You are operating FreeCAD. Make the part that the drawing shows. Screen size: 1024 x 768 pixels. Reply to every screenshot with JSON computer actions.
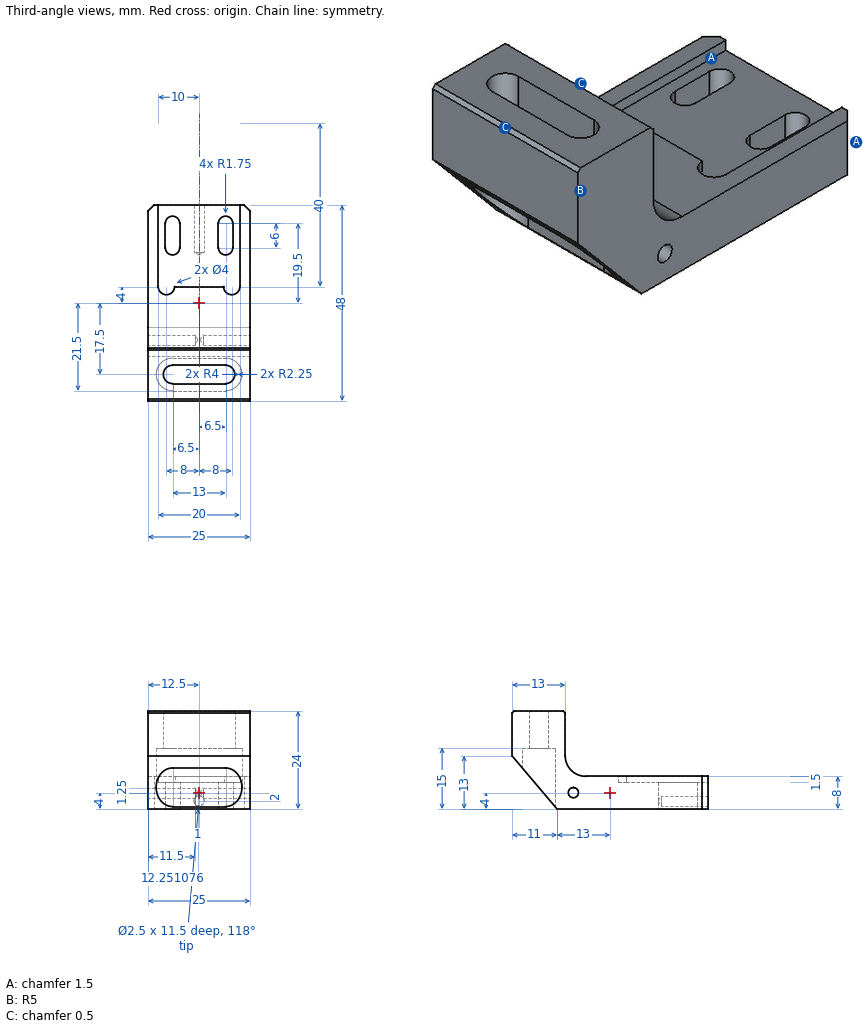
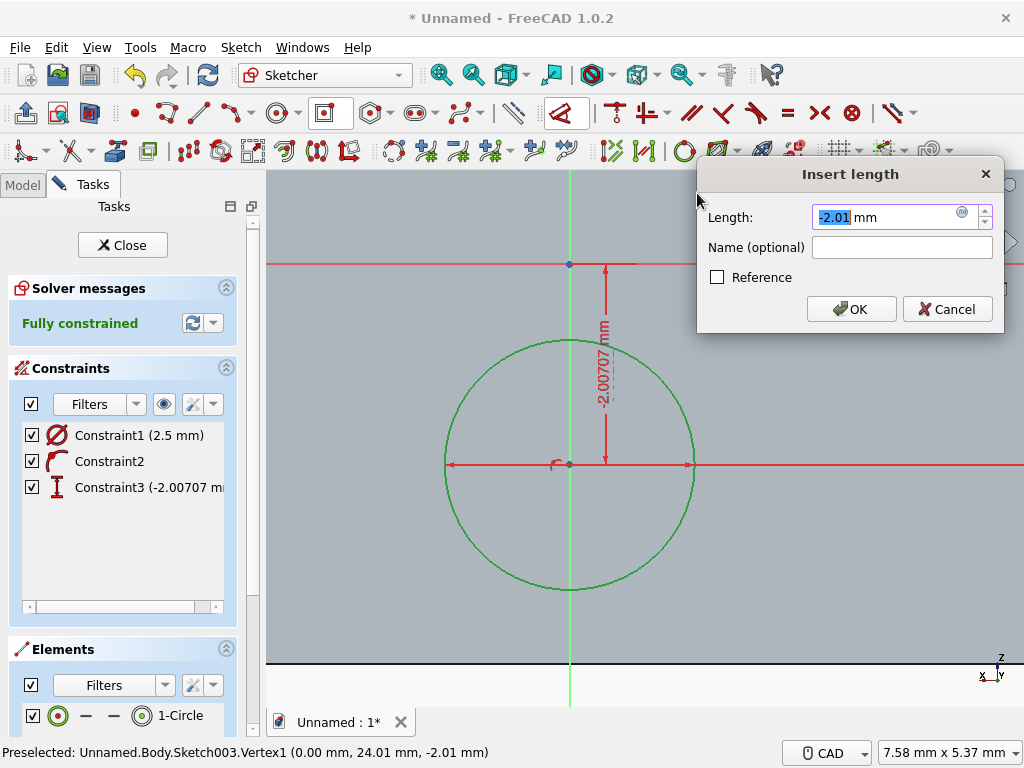
{"action": "type", "text": "-2"}
{"action": "key", "text": "Return"}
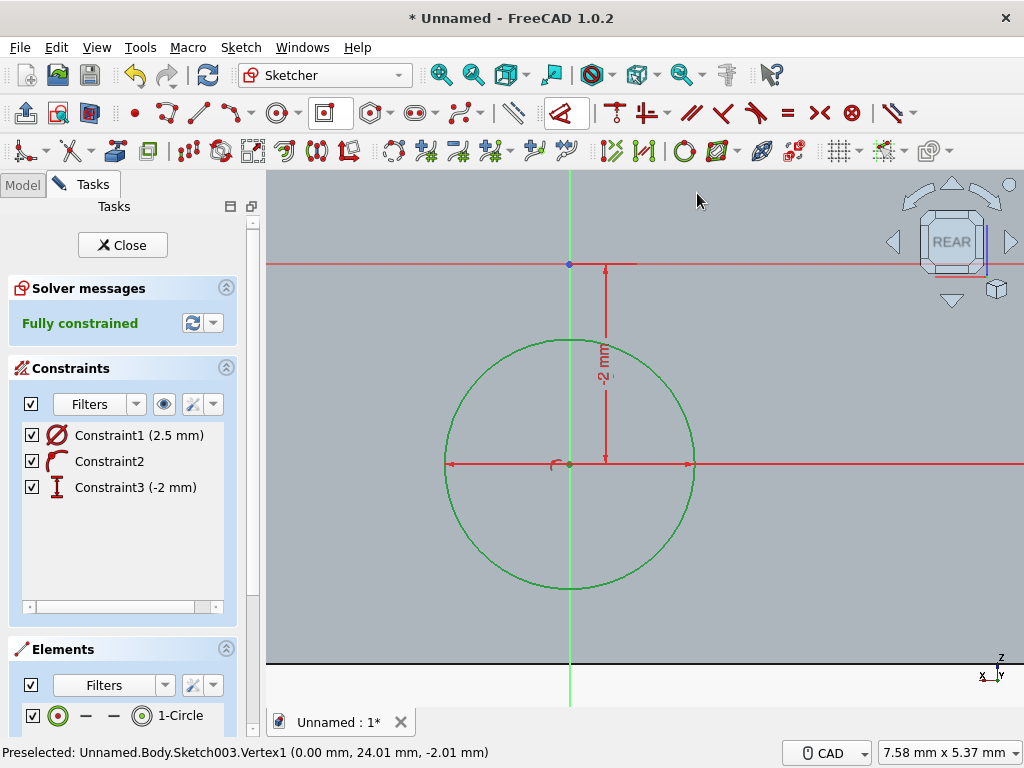
{"action": "left_click", "coordinate": [123, 245]}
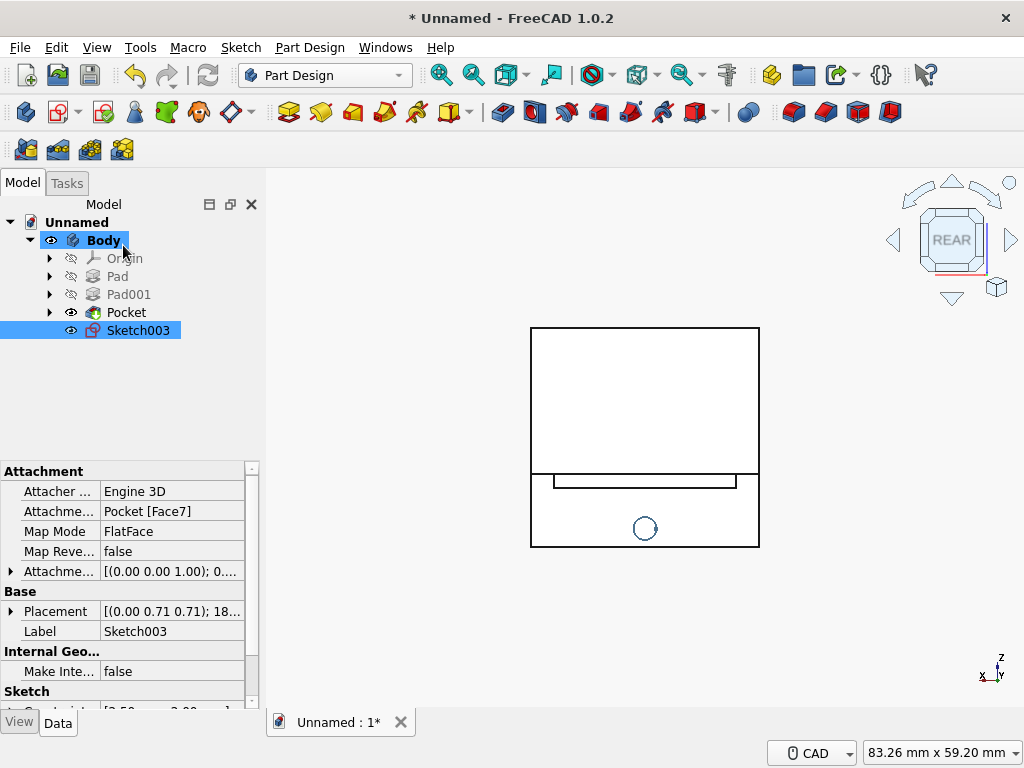
{"action": "left_click", "coordinate": [536, 112]}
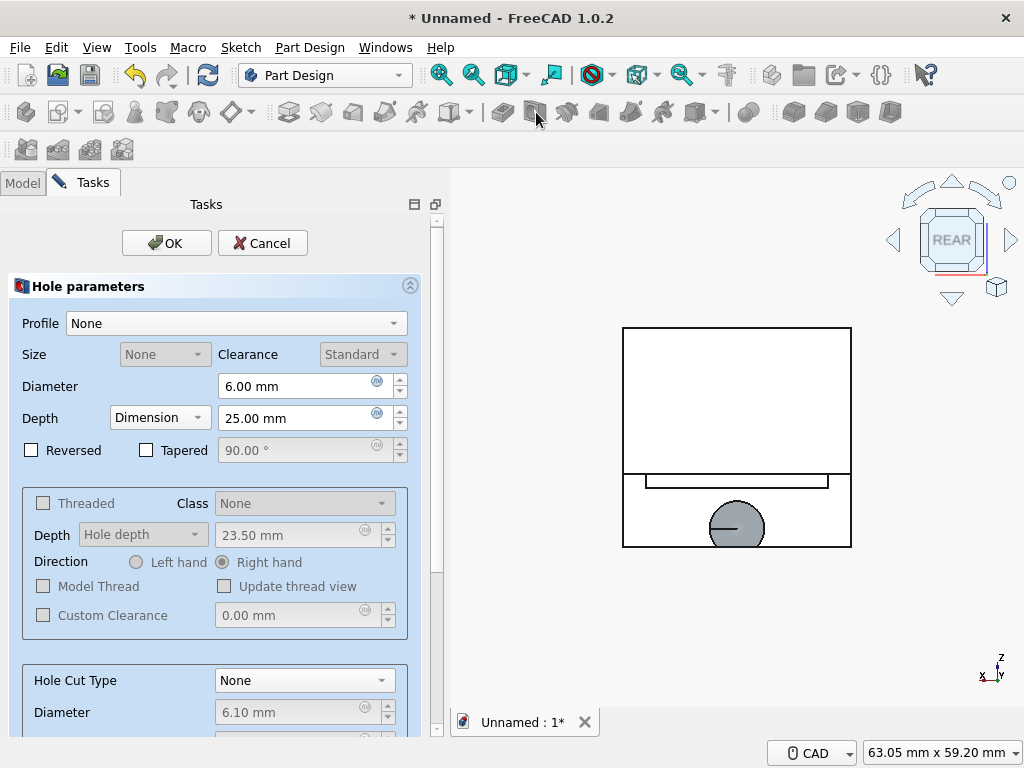
{"action": "triple_click", "coordinate": [305, 386]}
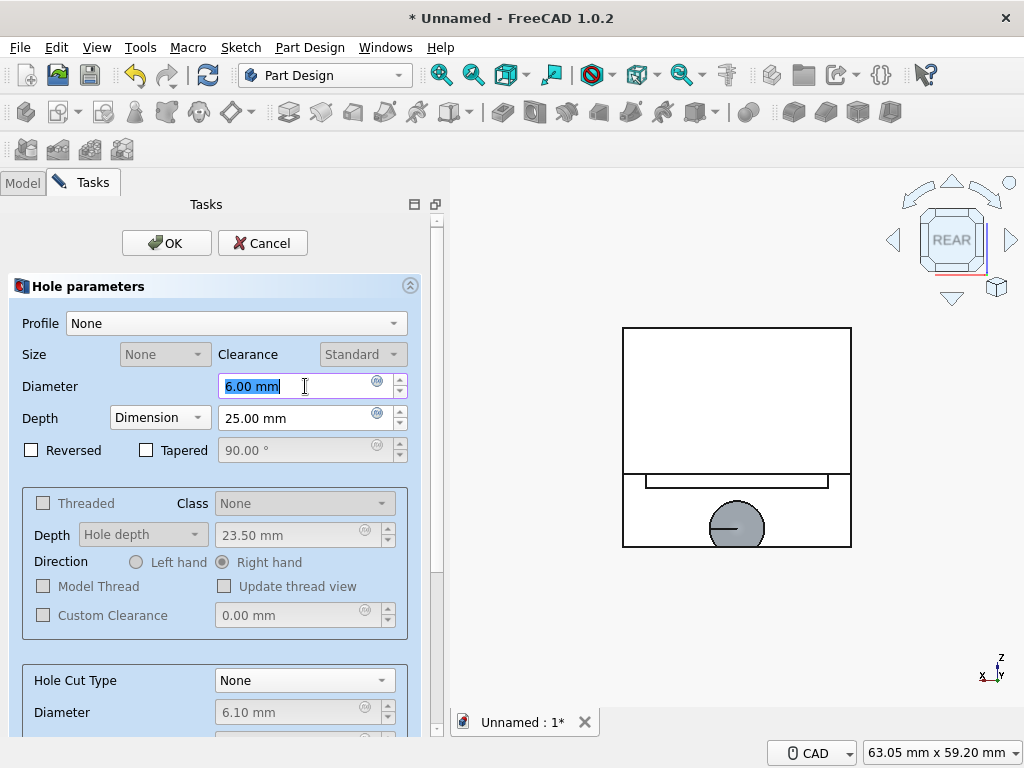
{"action": "type", "text": "2.5"}
{"action": "key", "text": "Tab"}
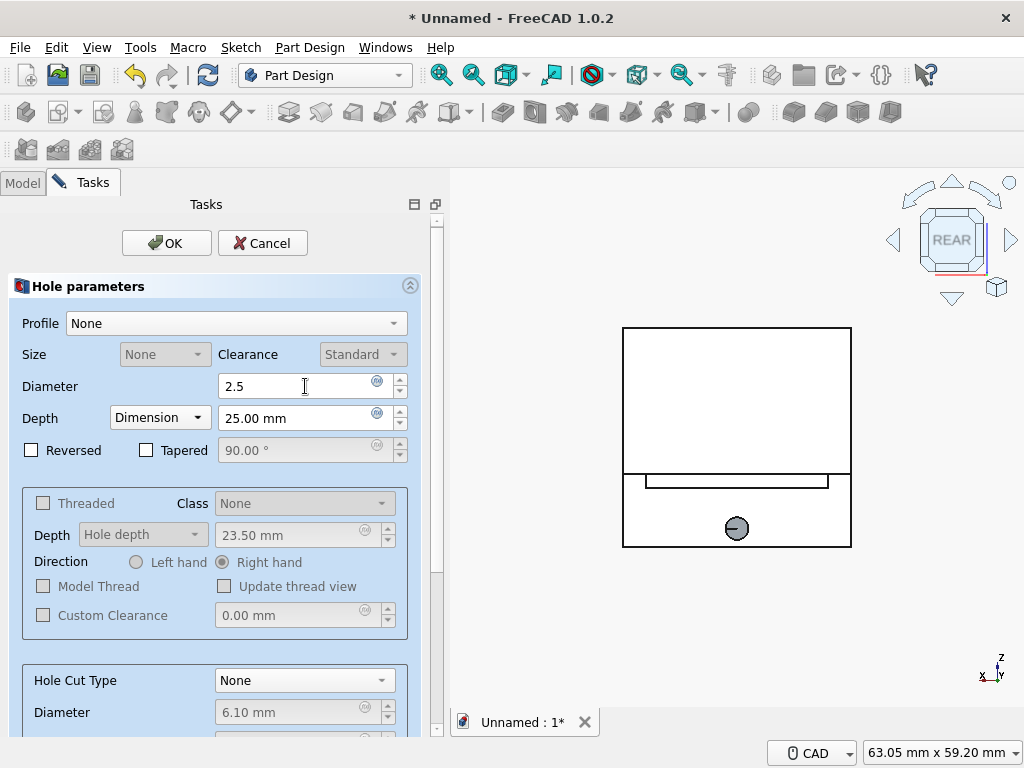
{"action": "triple_click", "coordinate": [305, 418]}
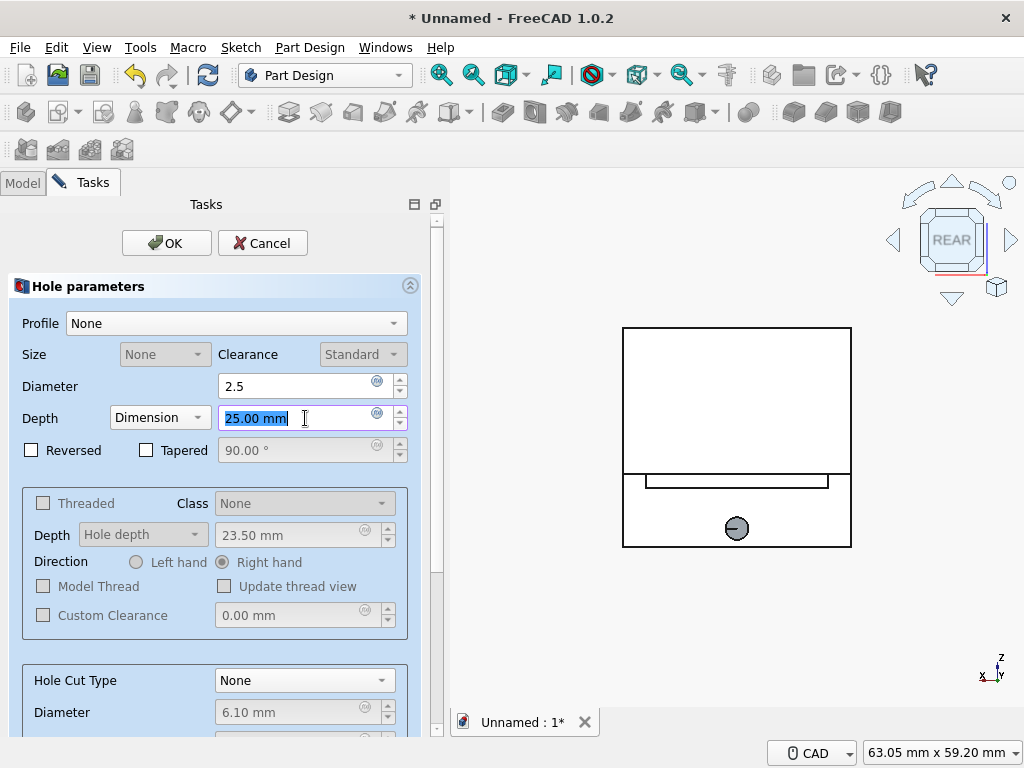
{"action": "type", "text": "11.5"}
{"action": "key", "text": "Tab"}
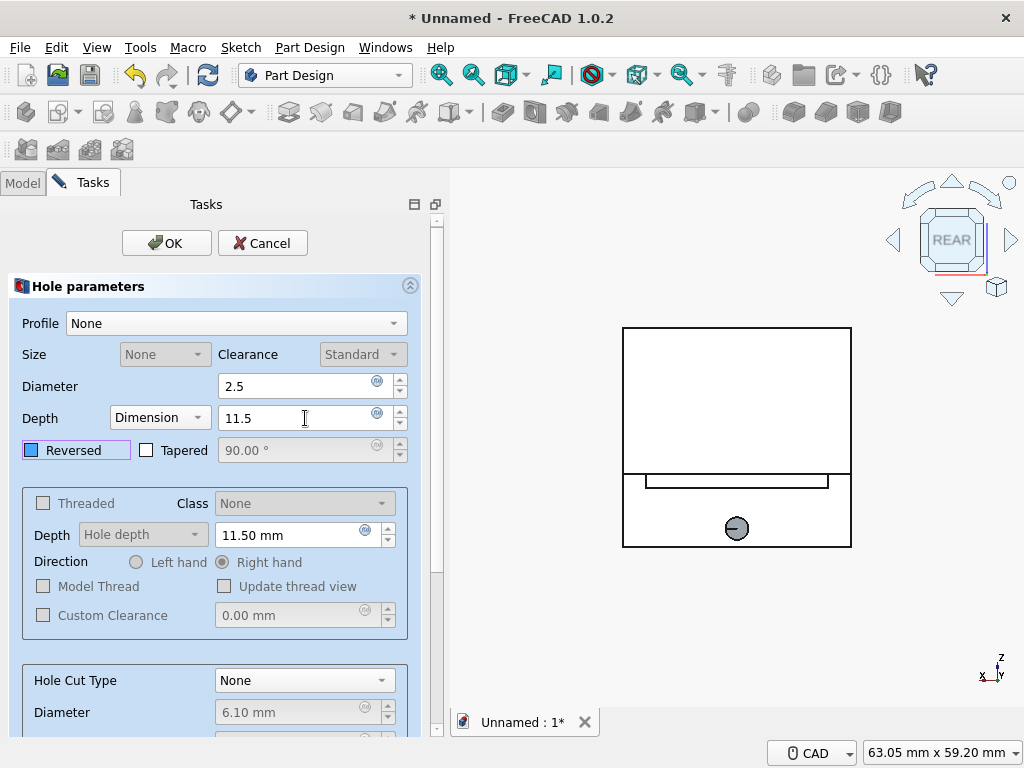
{"action": "left_click", "coordinate": [167, 243]}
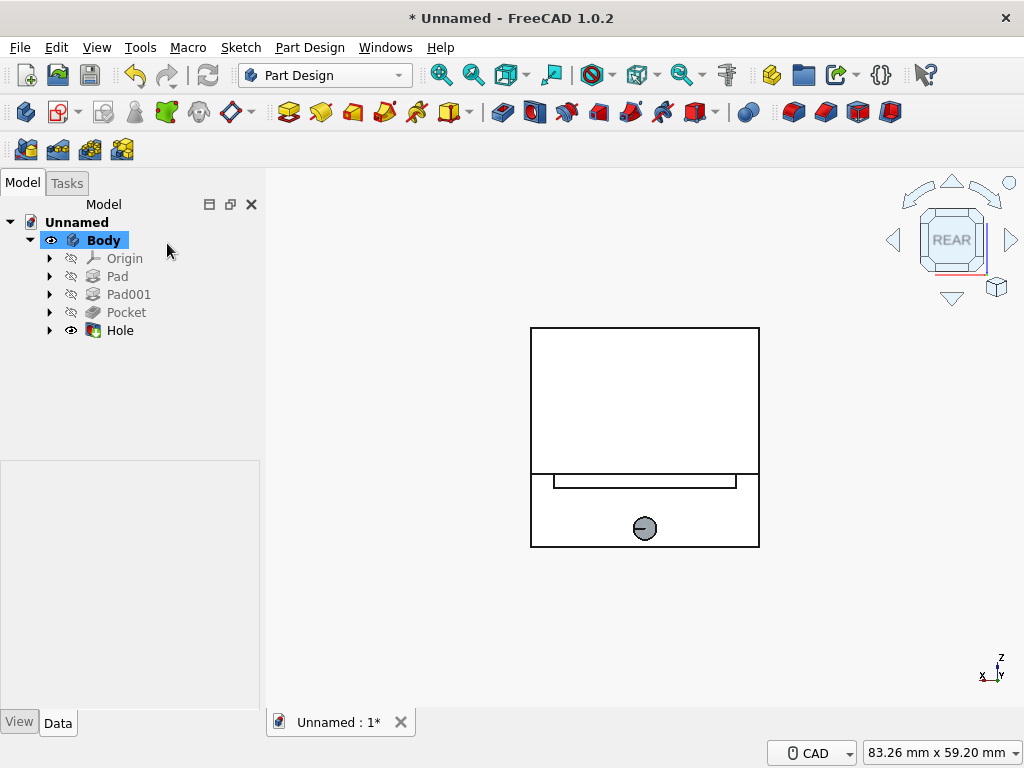
{"action": "left_click", "coordinate": [442, 76]}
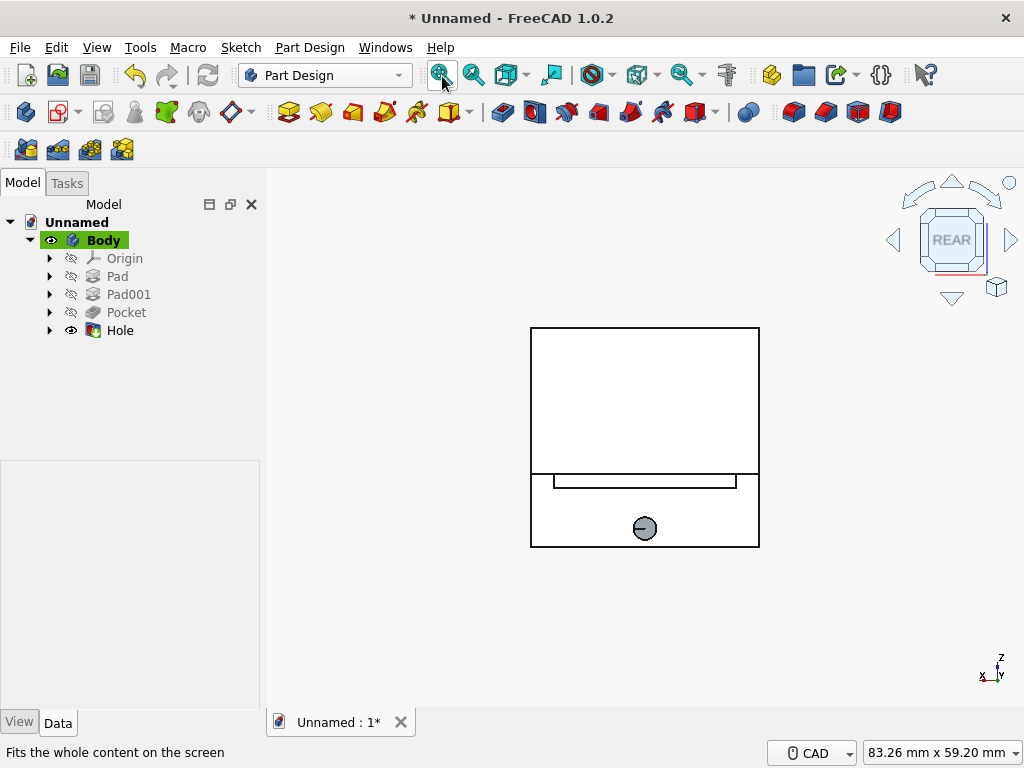
{"action": "left_click", "coordinate": [759, 509]}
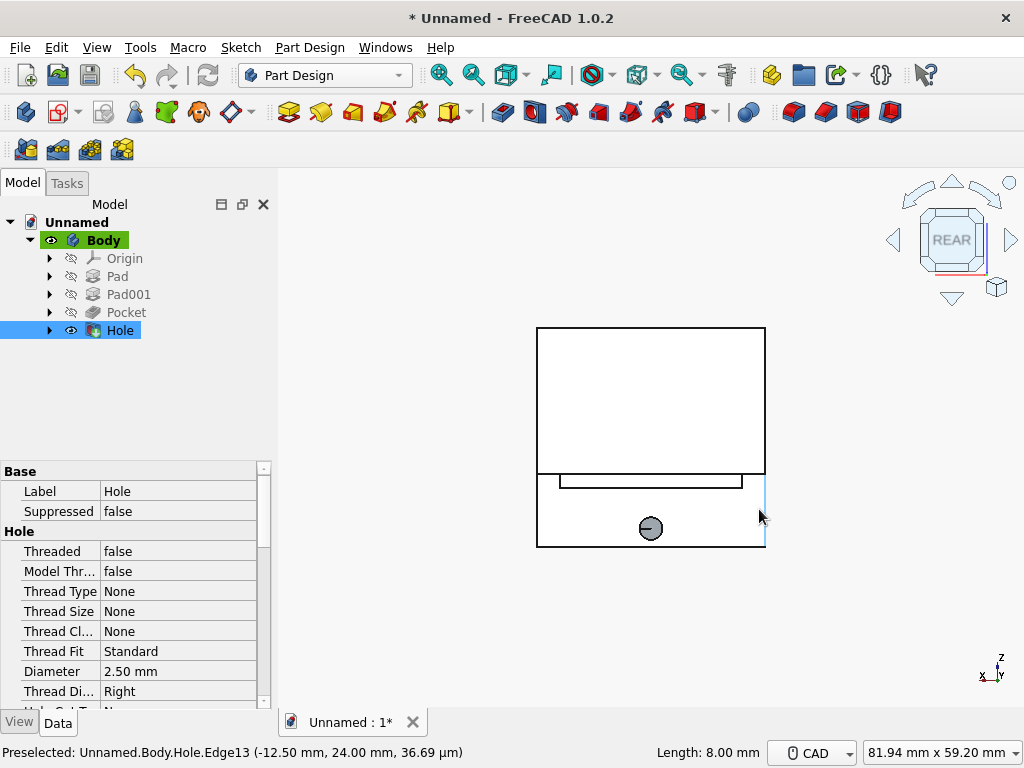
{"action": "key", "text": "0"}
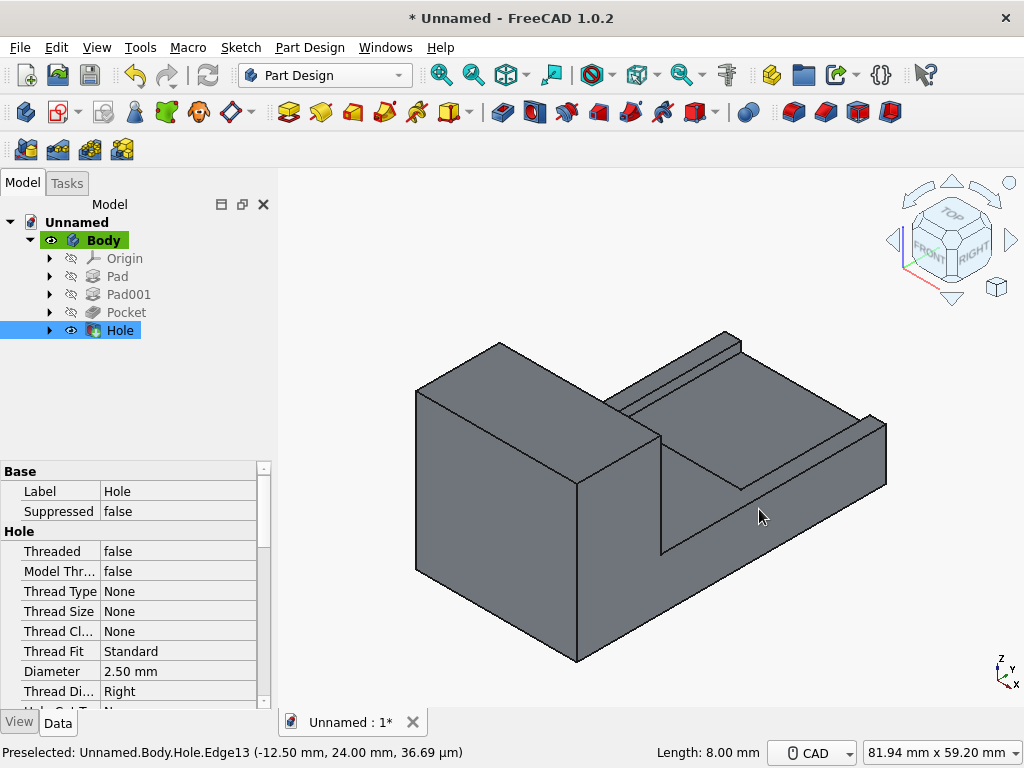
{"action": "key", "text": "2"}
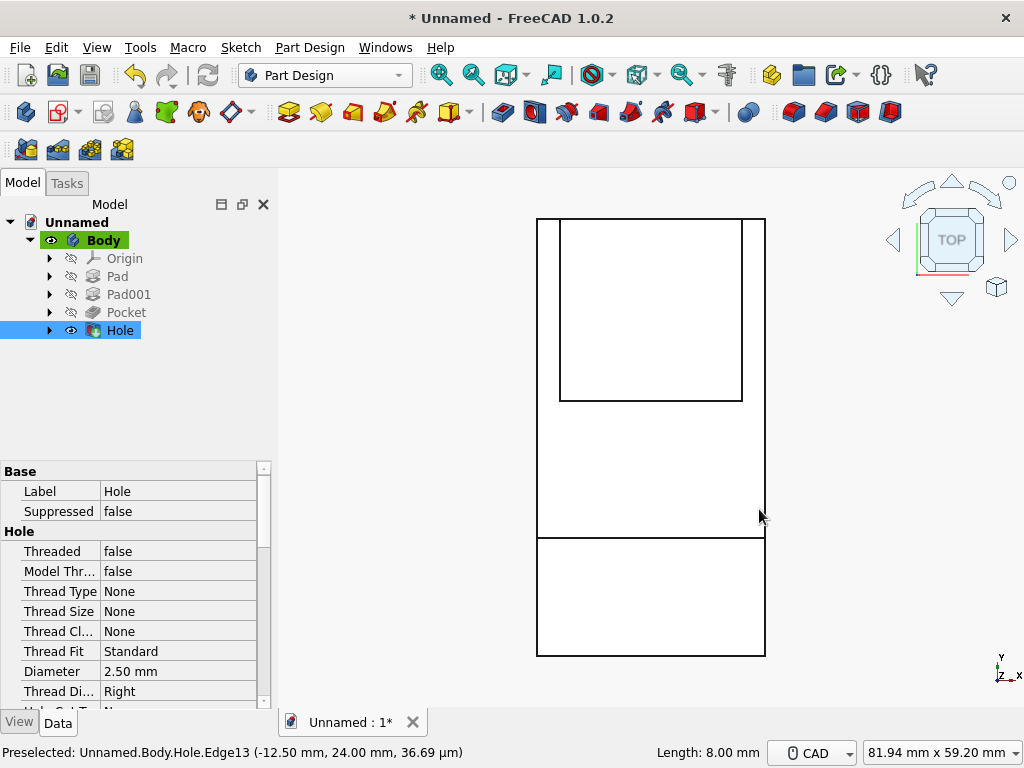
{"action": "key", "text": "1"}